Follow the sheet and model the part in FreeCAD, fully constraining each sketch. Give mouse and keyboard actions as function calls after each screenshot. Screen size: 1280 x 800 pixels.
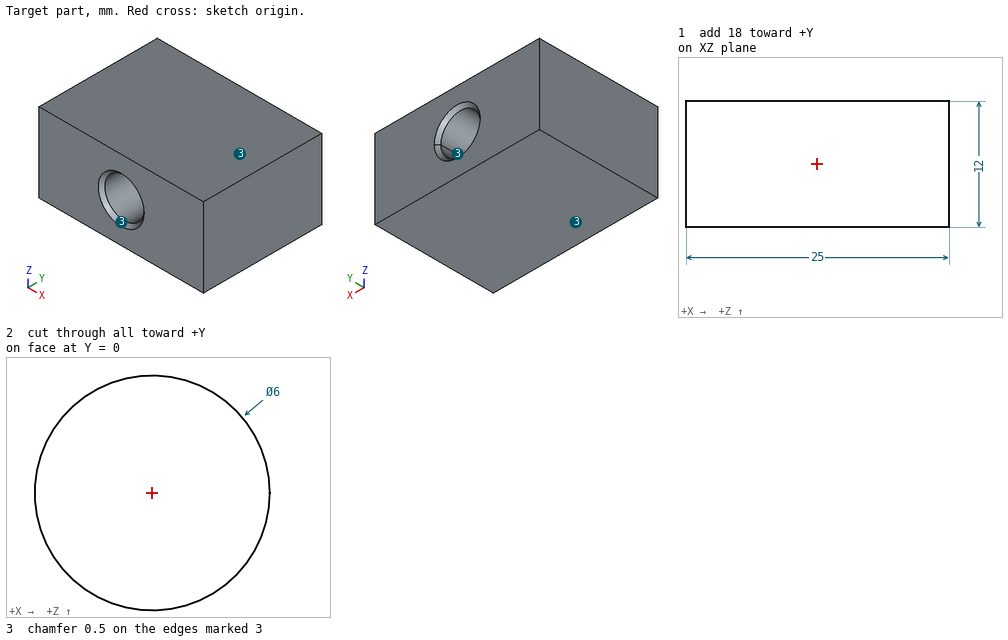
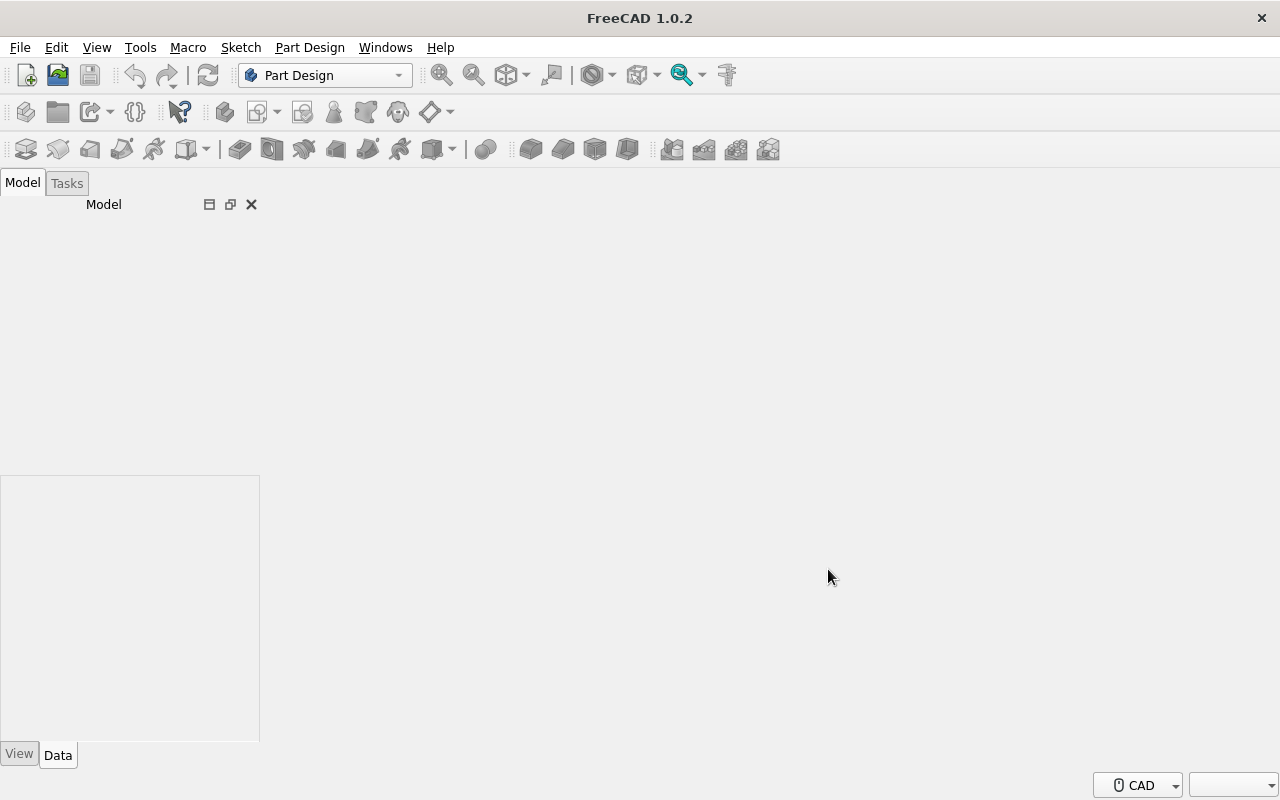
key(ctrl+n)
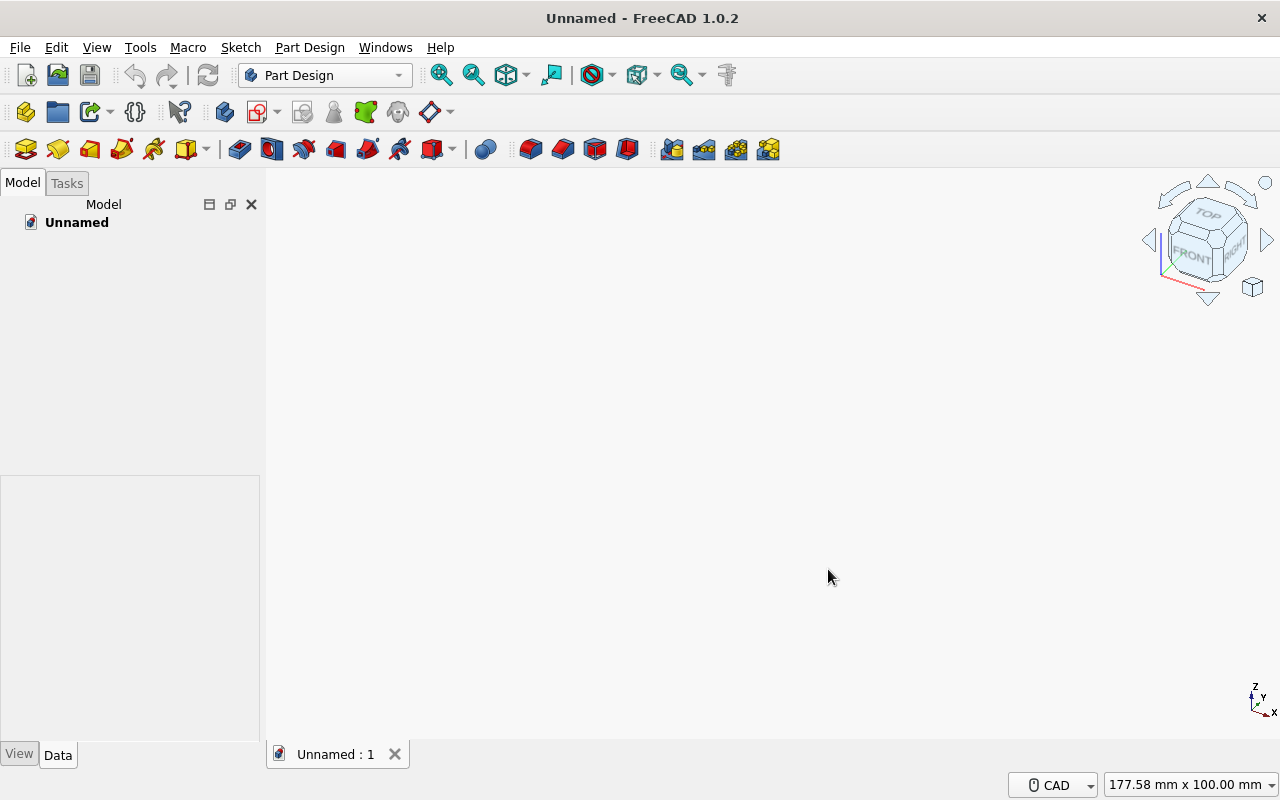
click(258, 112)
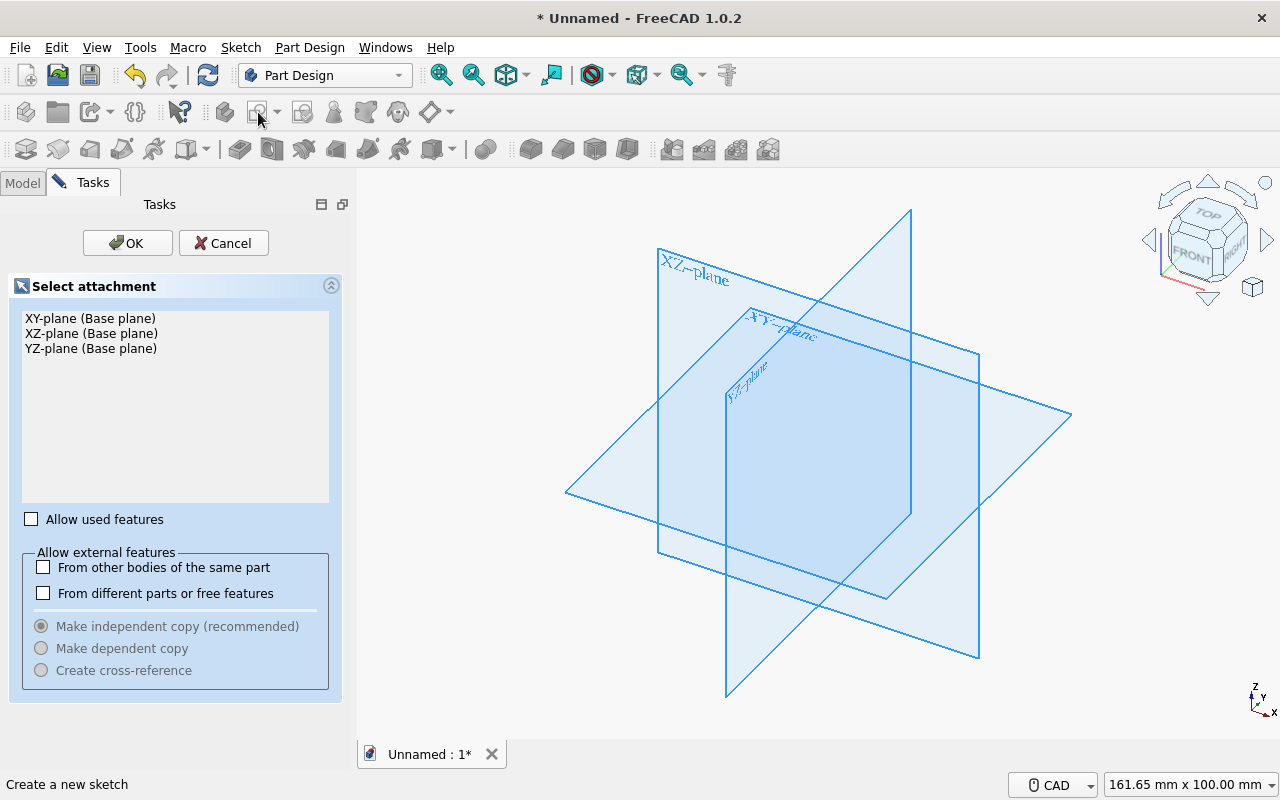
click(82, 334)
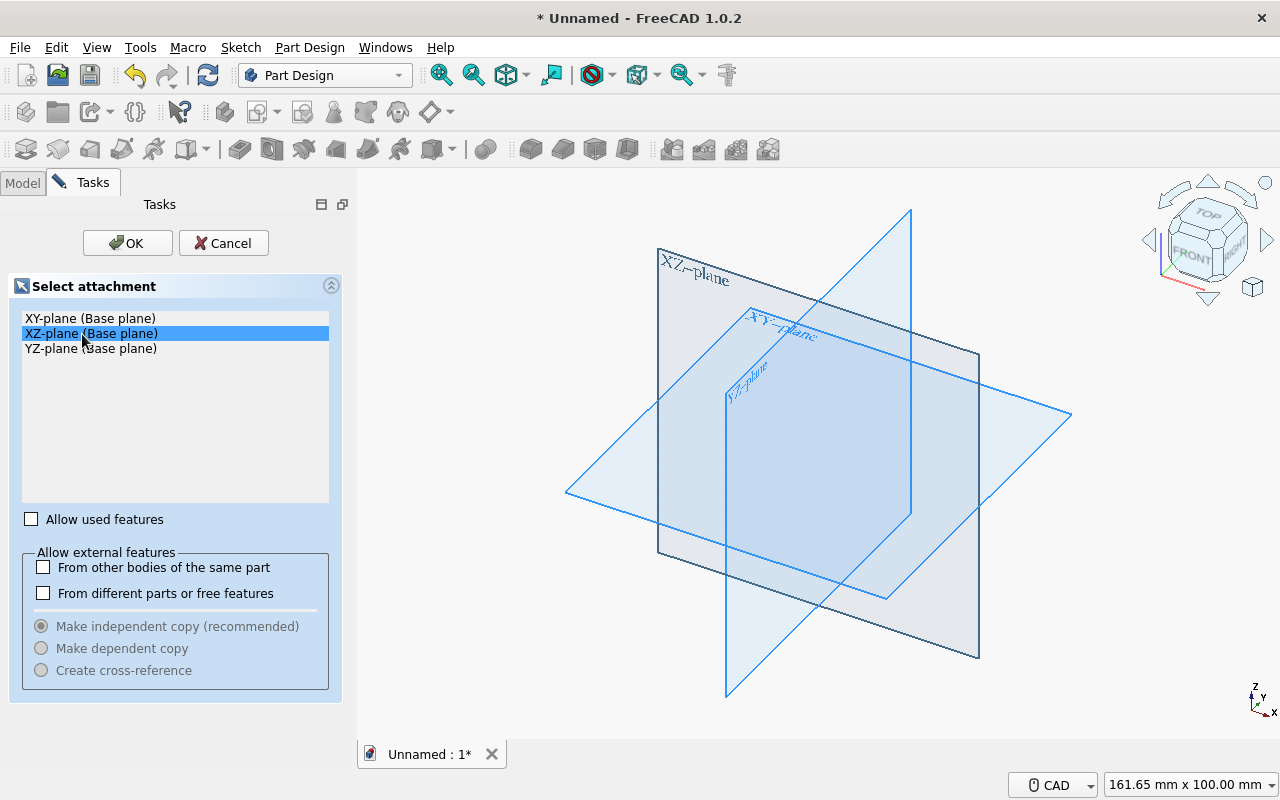
click(128, 243)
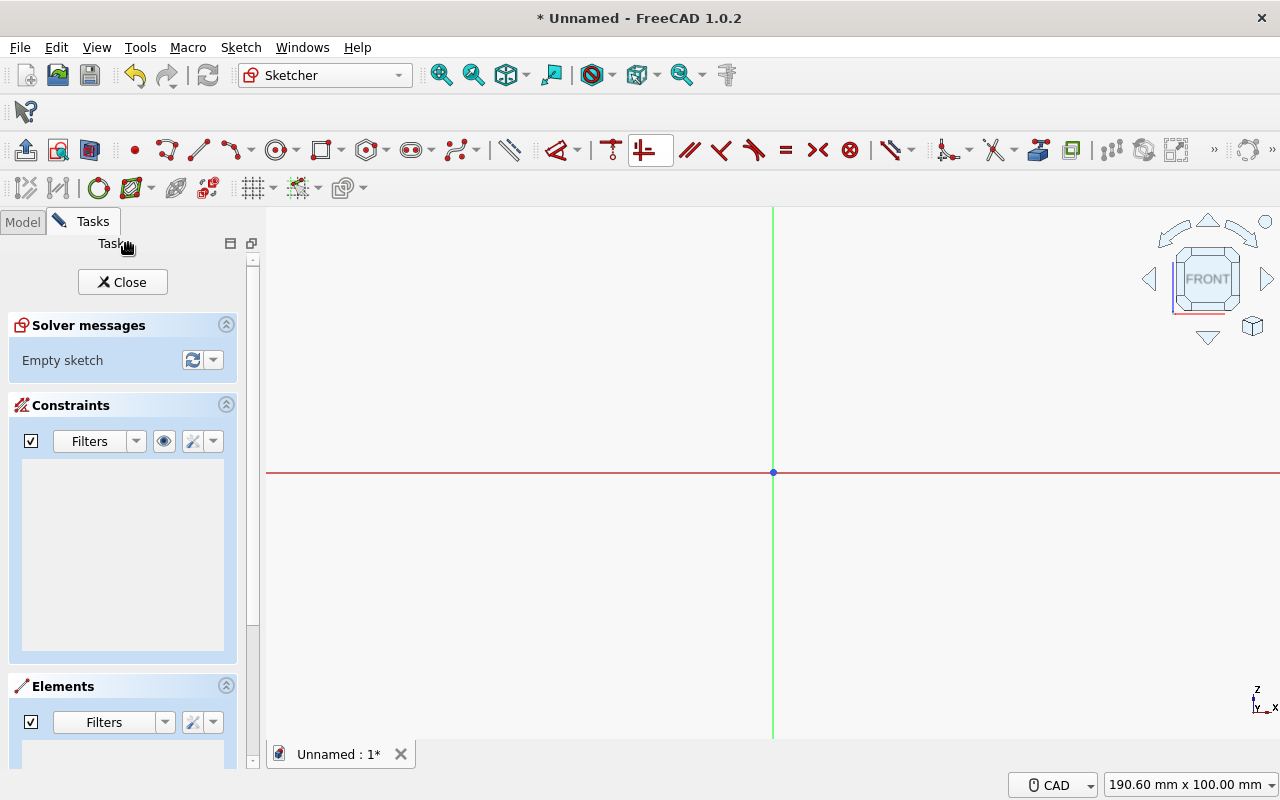
scroll(795, 473, up, 7)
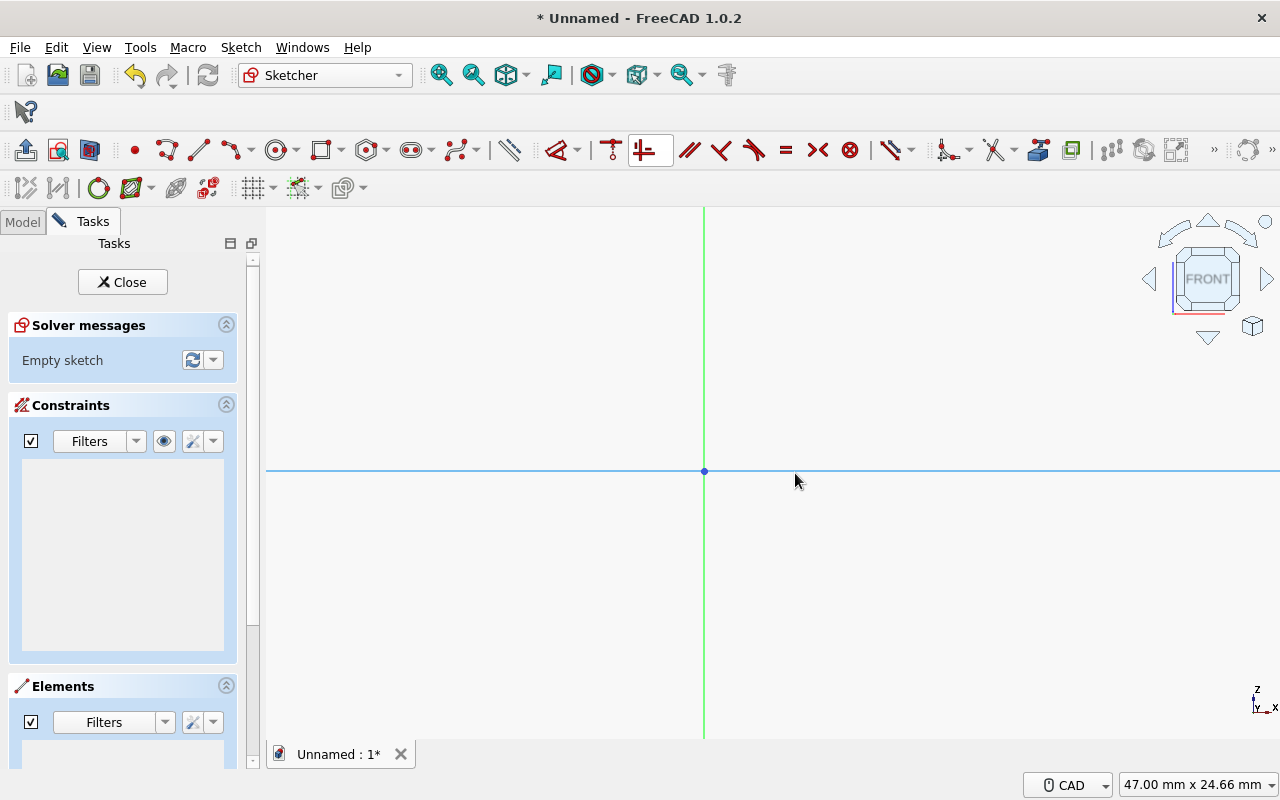
click(344, 150)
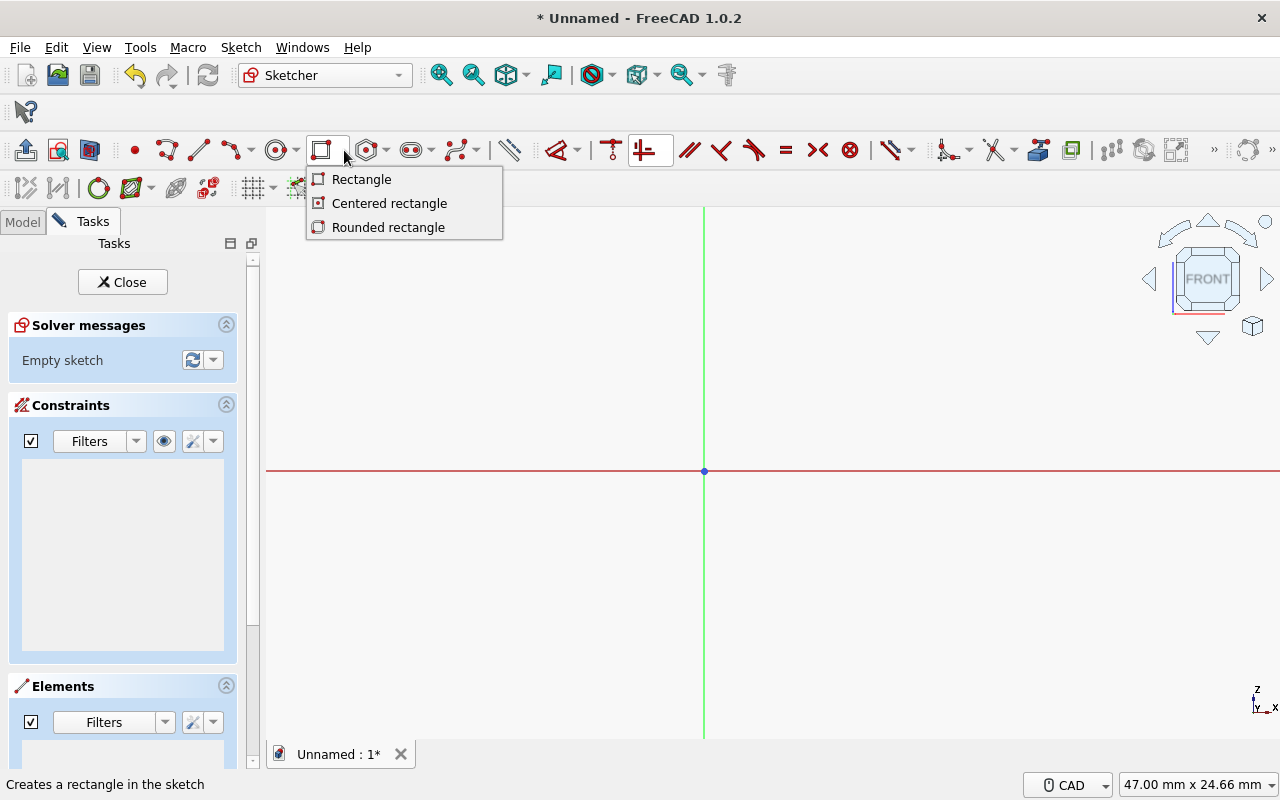
click(404, 203)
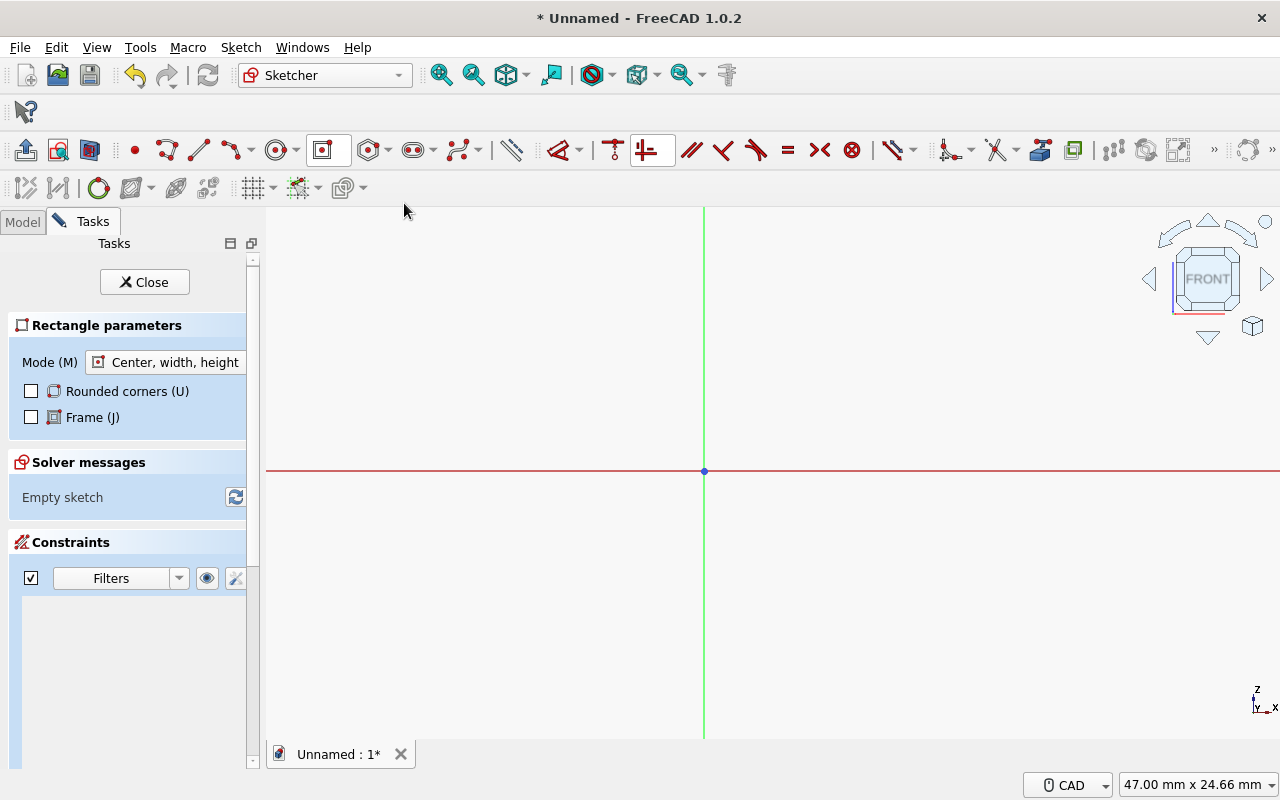
click(704, 471)
move(974, 342)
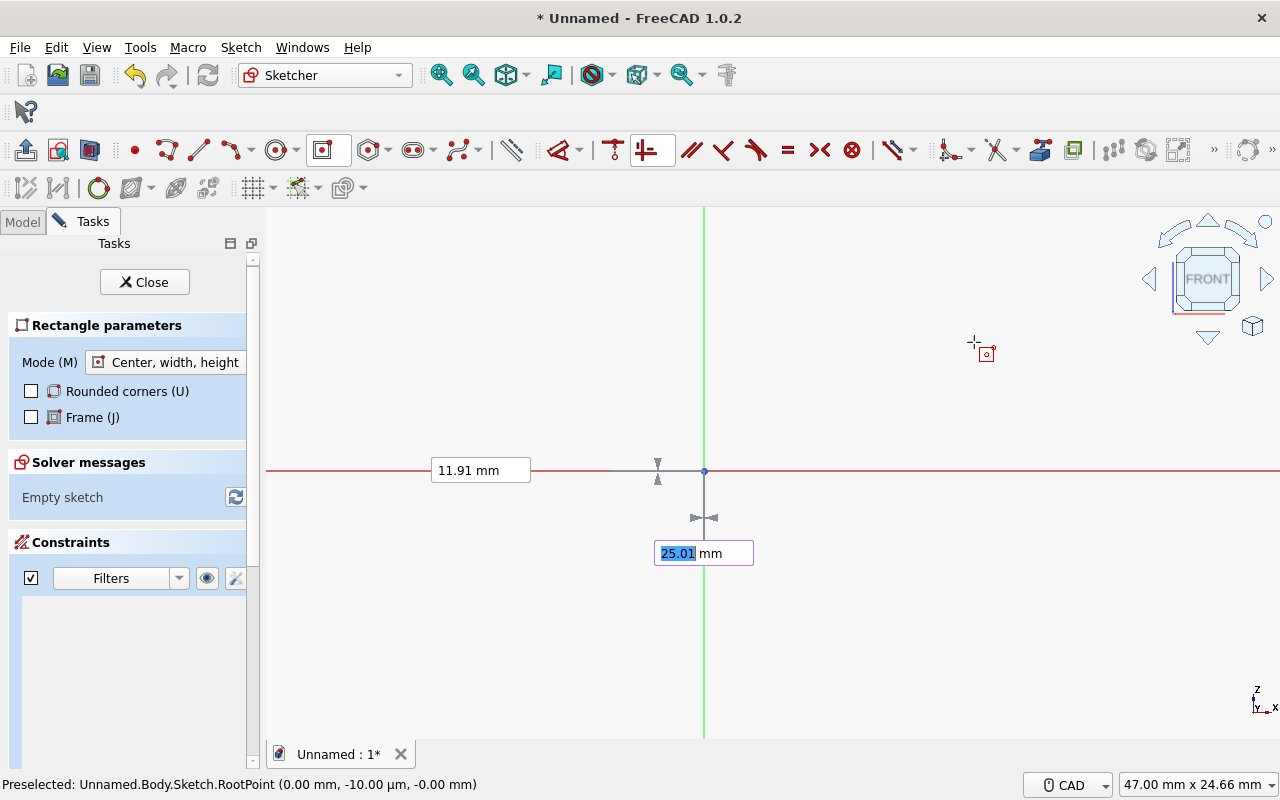
text(25)
key(Tab)
text(12)
key(Return)
key(Escape)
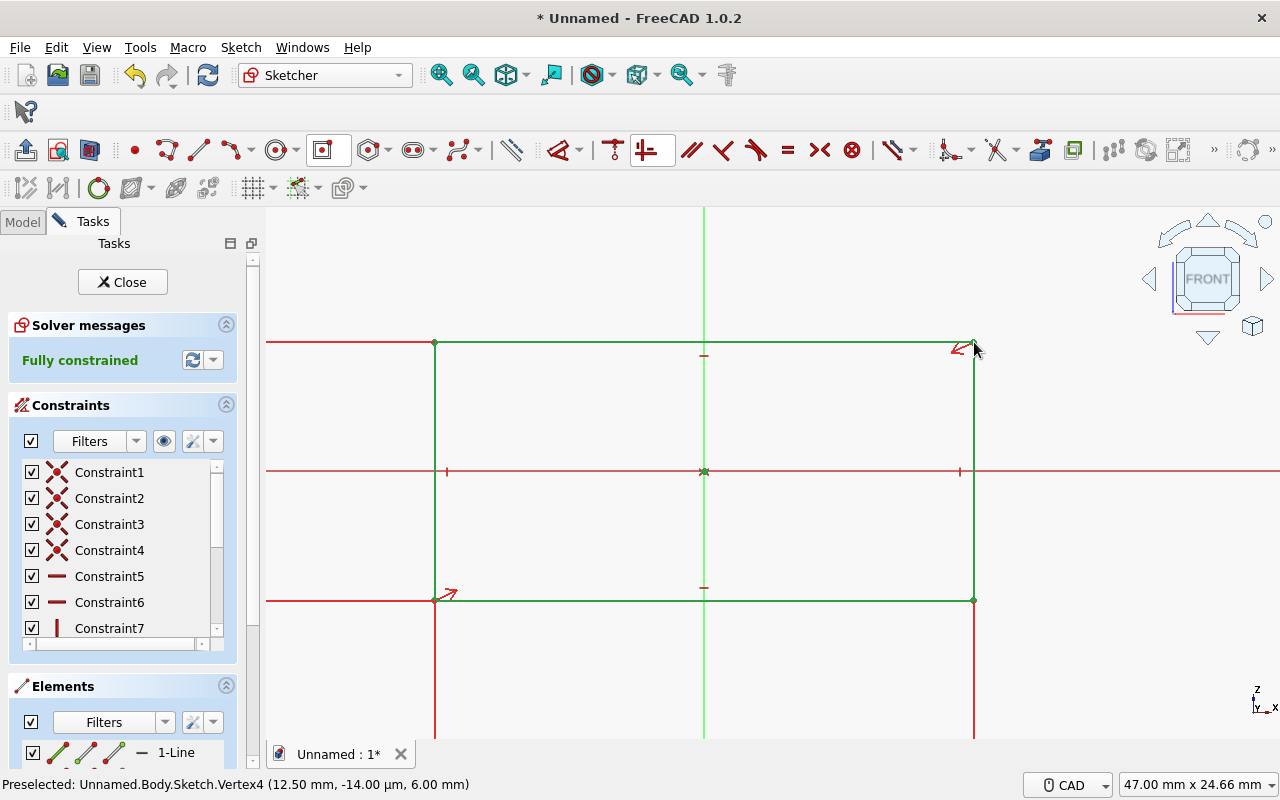
click(123, 282)